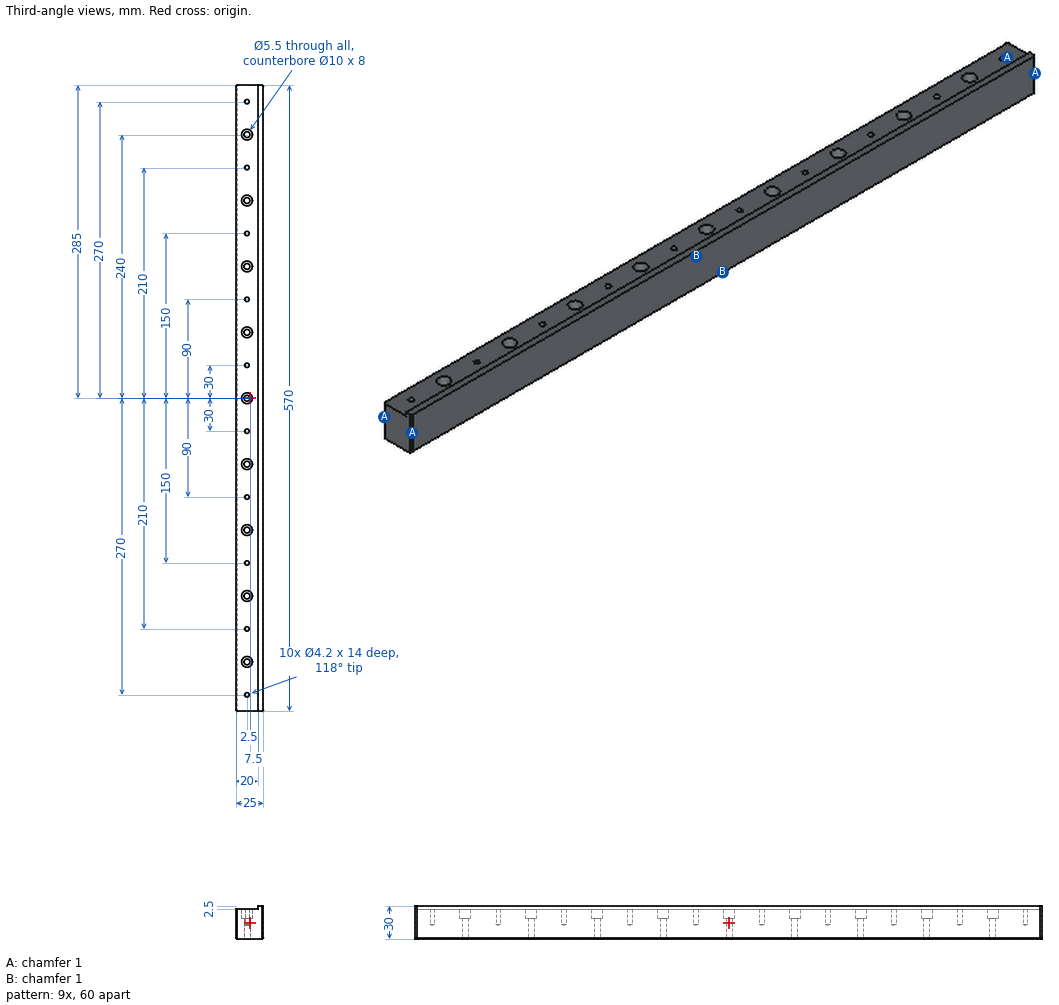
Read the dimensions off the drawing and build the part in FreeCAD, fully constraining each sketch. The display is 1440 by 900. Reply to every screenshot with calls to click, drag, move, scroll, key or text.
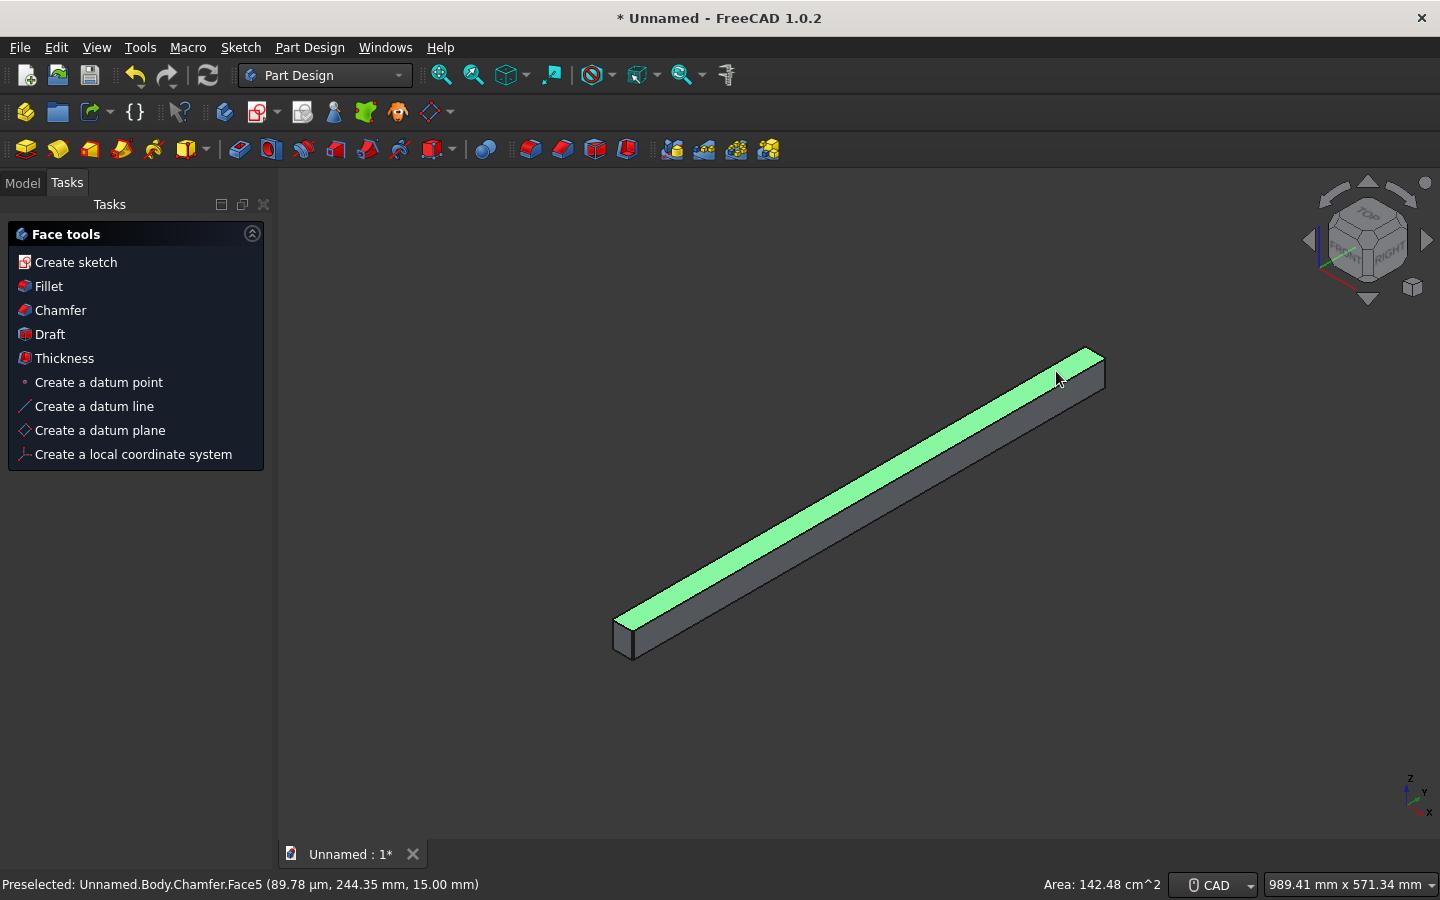
click(258, 112)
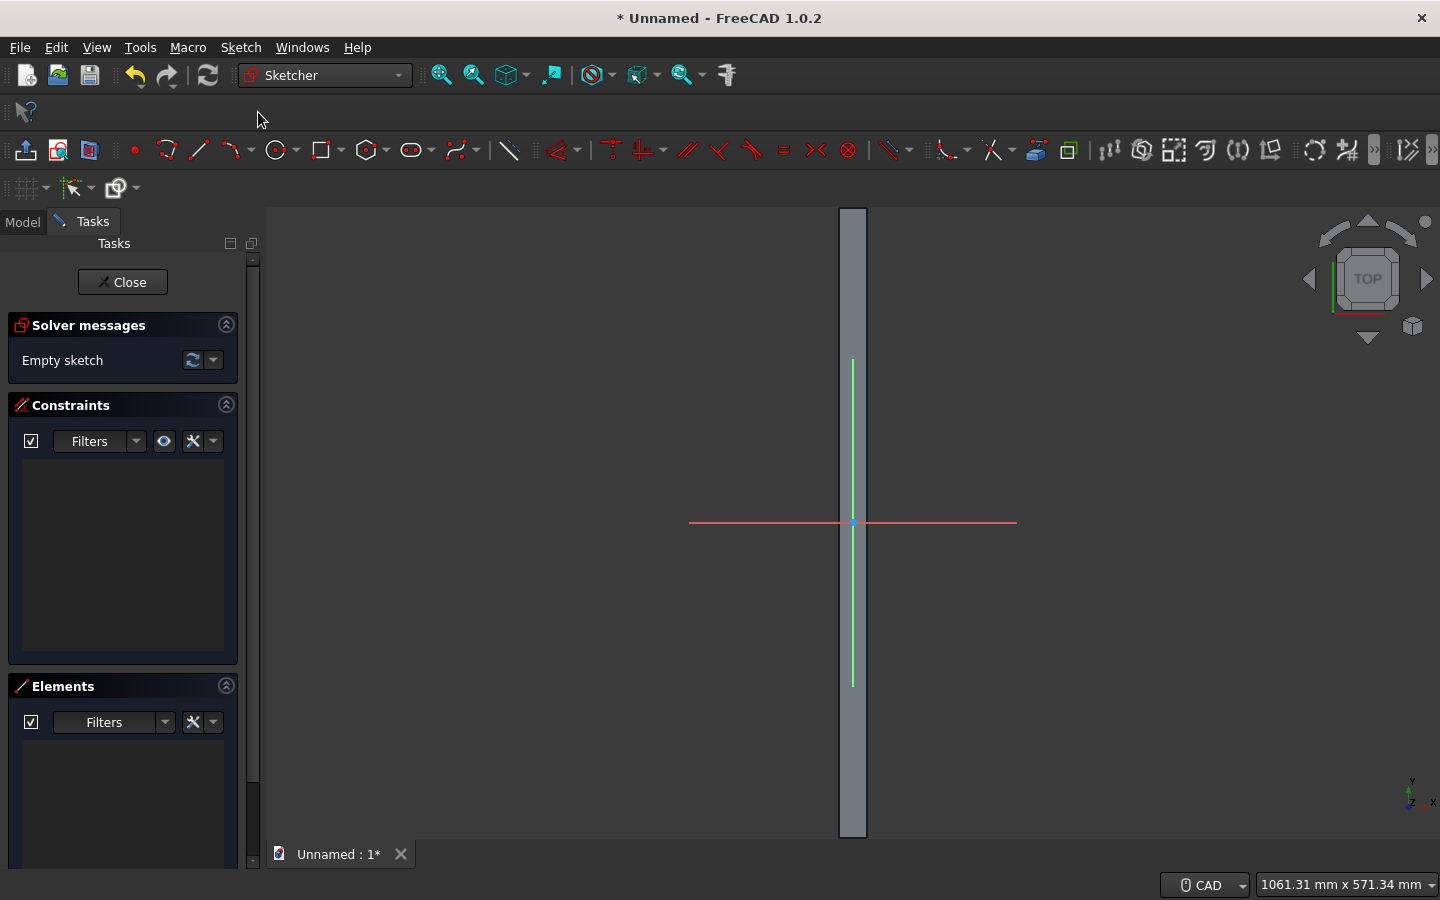
scroll(651, 523, down, 2)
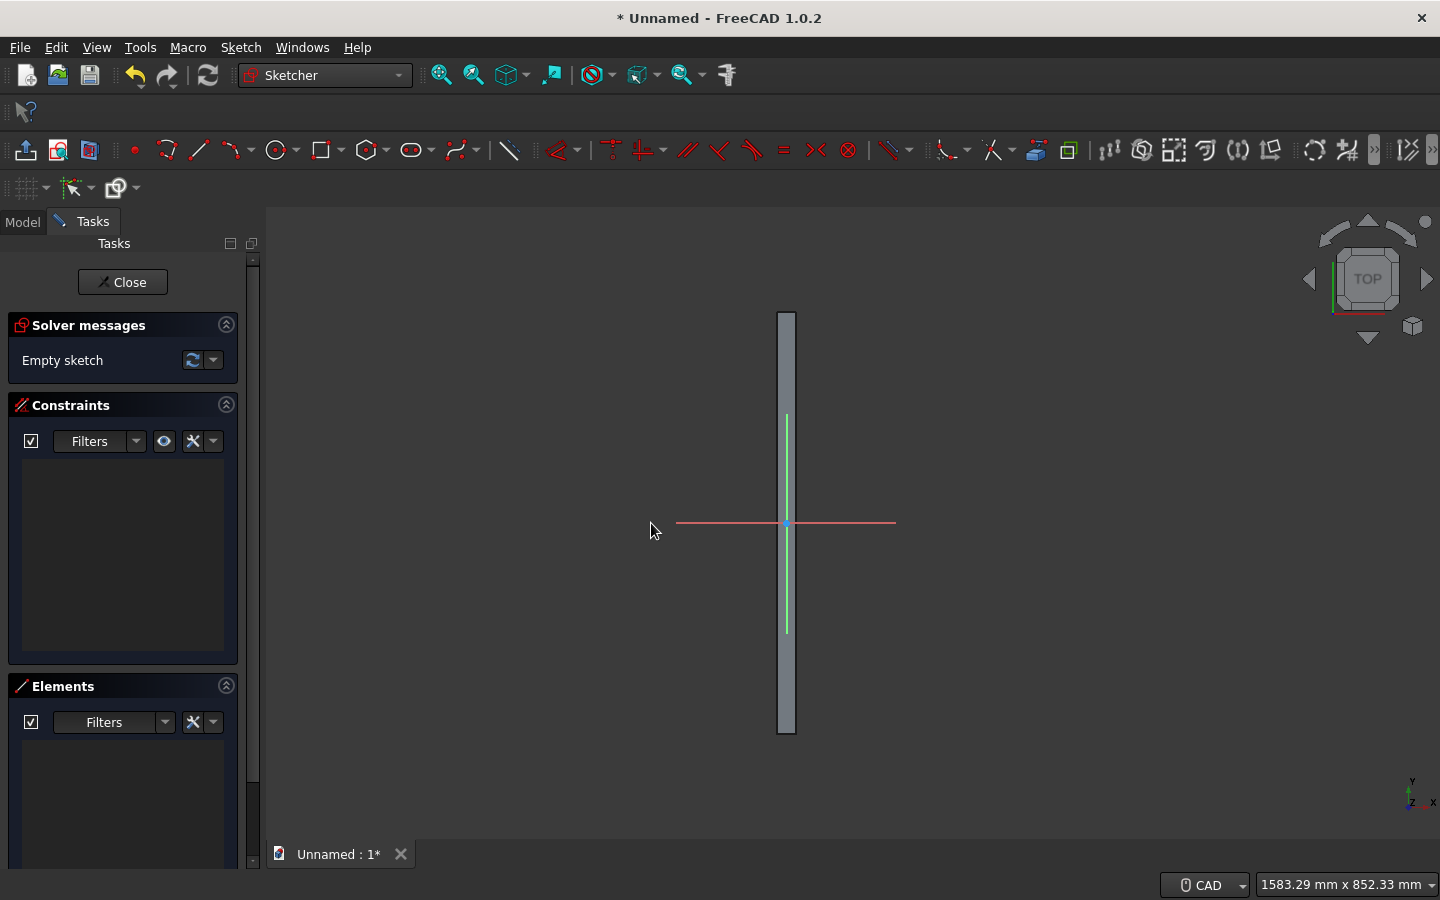
key(g)
key(r)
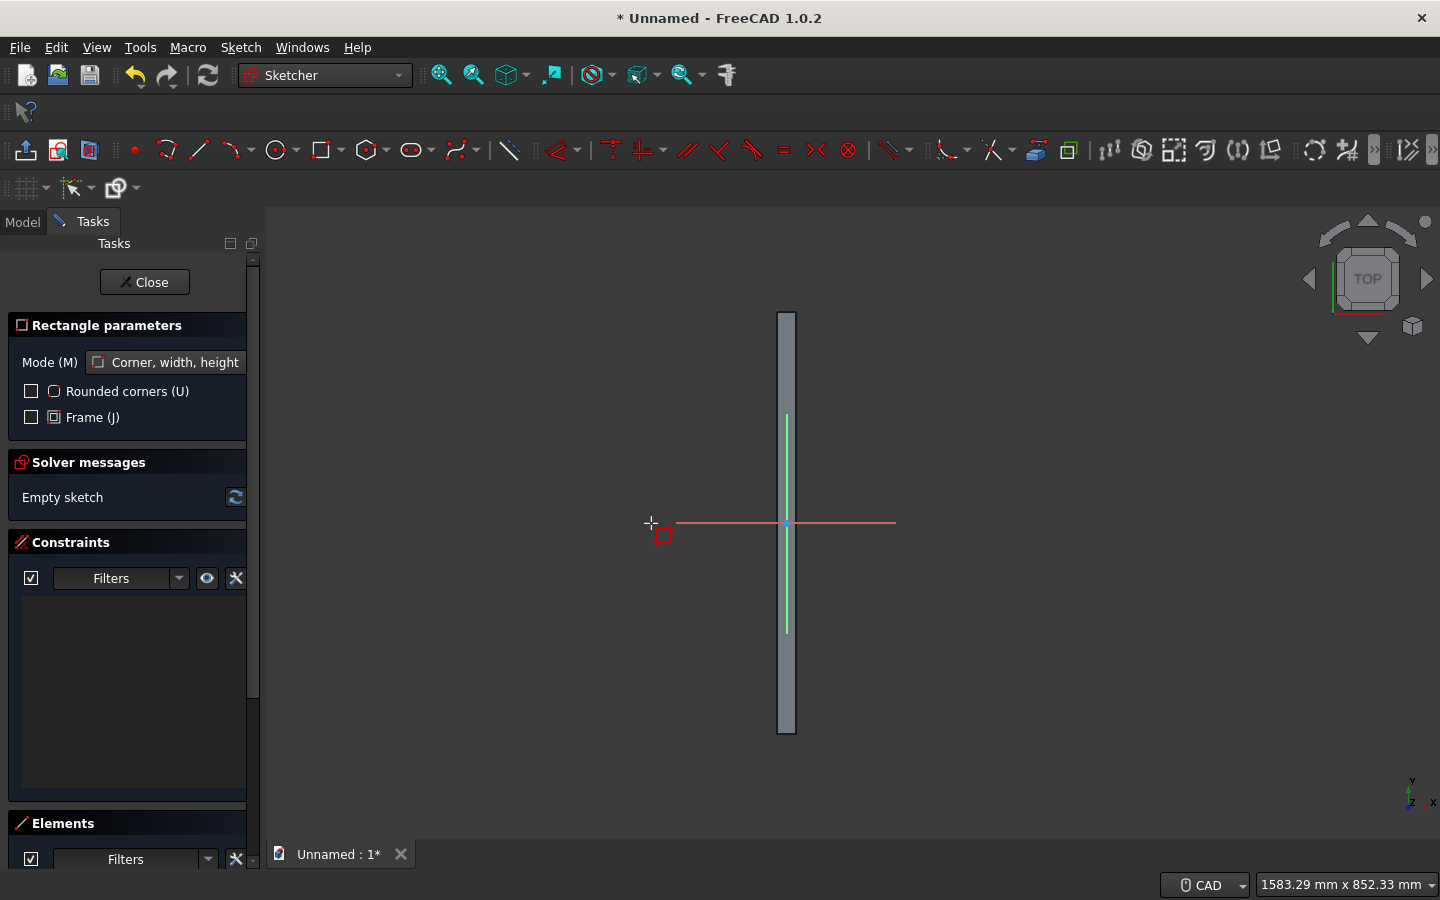
scroll(777, 312, up, 3)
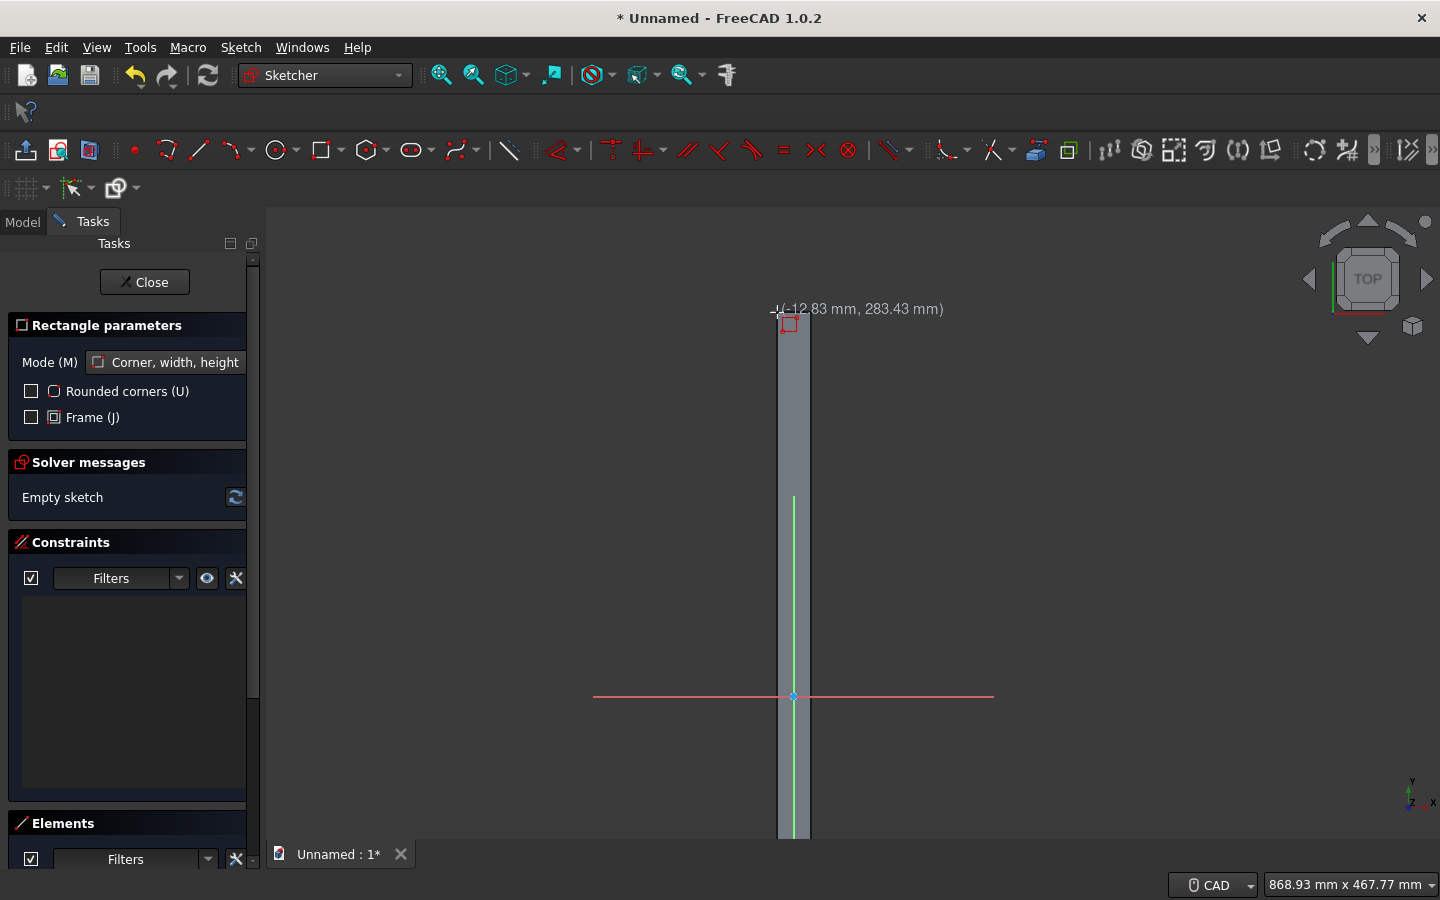
click(777, 312)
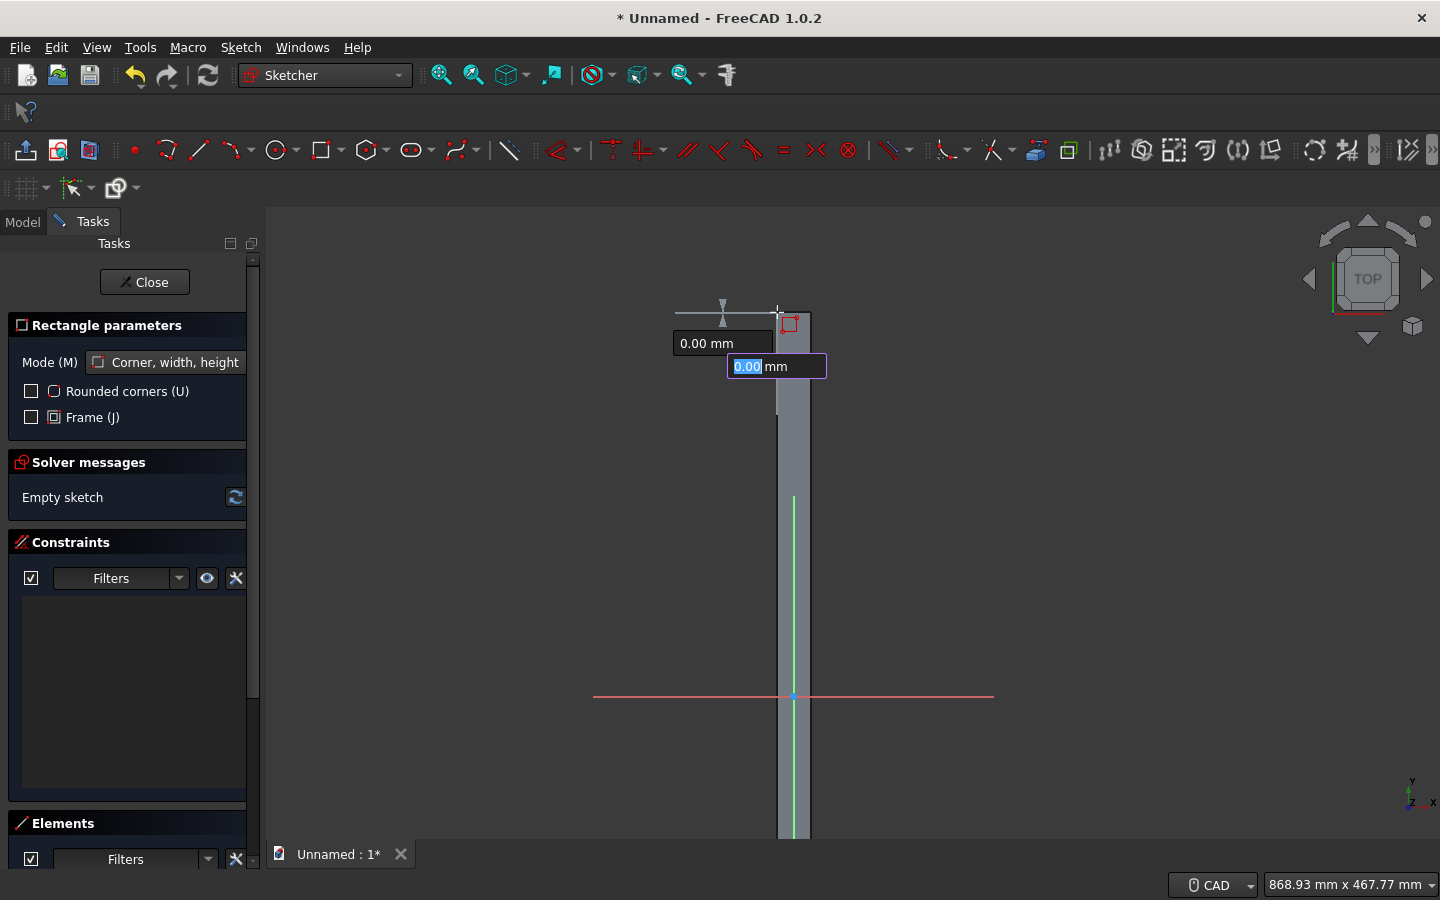
scroll(777, 312, down, 3)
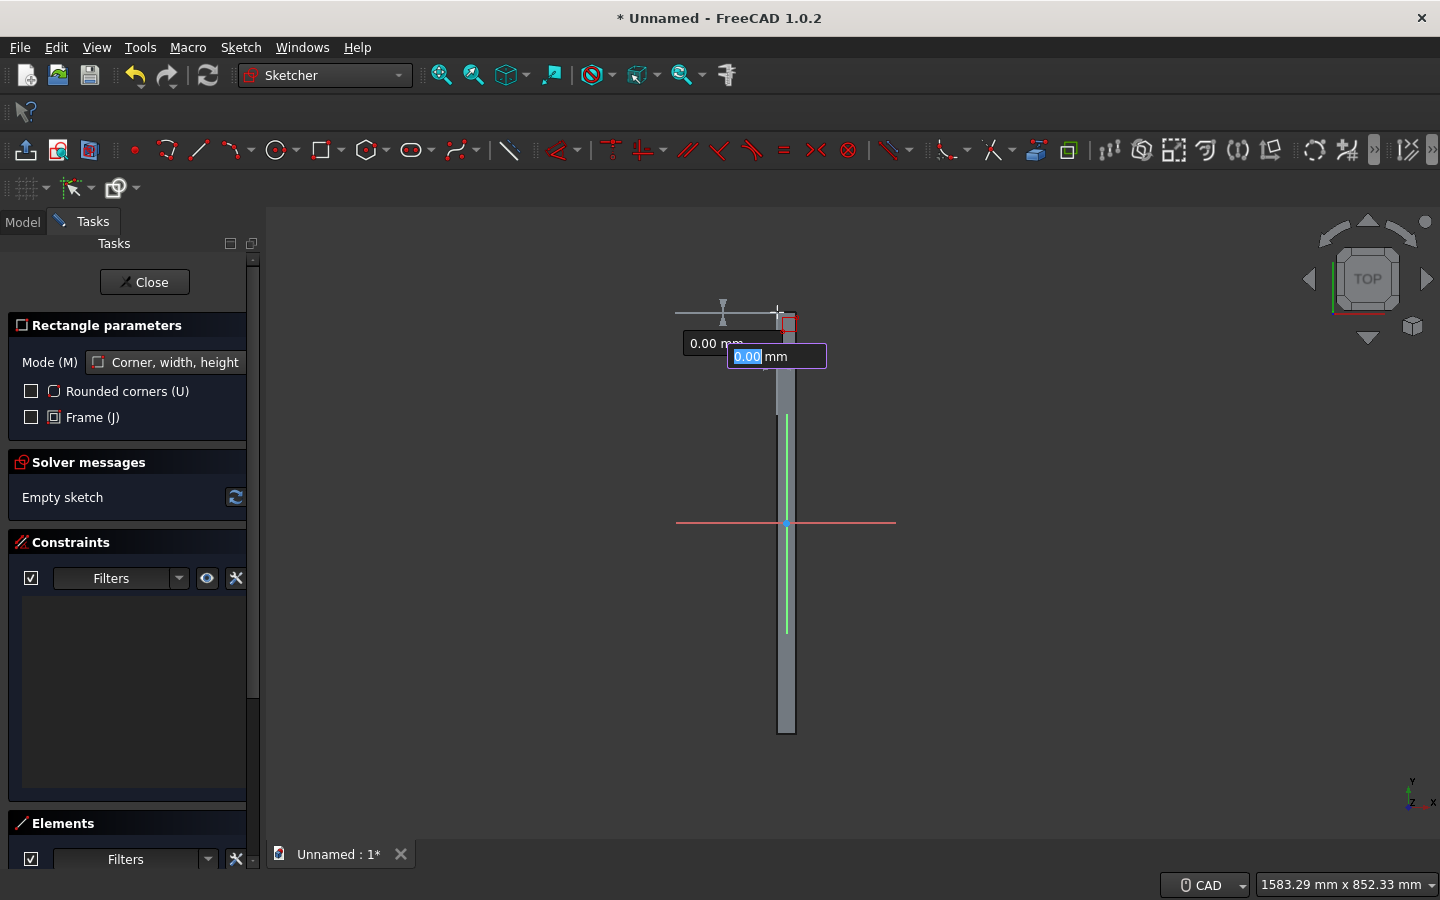
scroll(792, 734, up, 6)